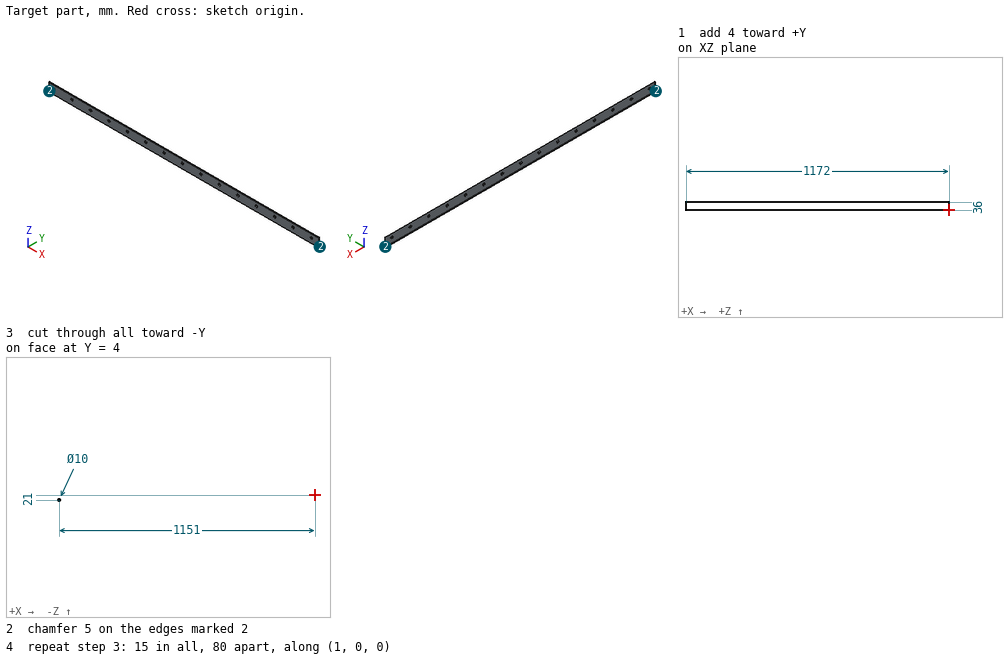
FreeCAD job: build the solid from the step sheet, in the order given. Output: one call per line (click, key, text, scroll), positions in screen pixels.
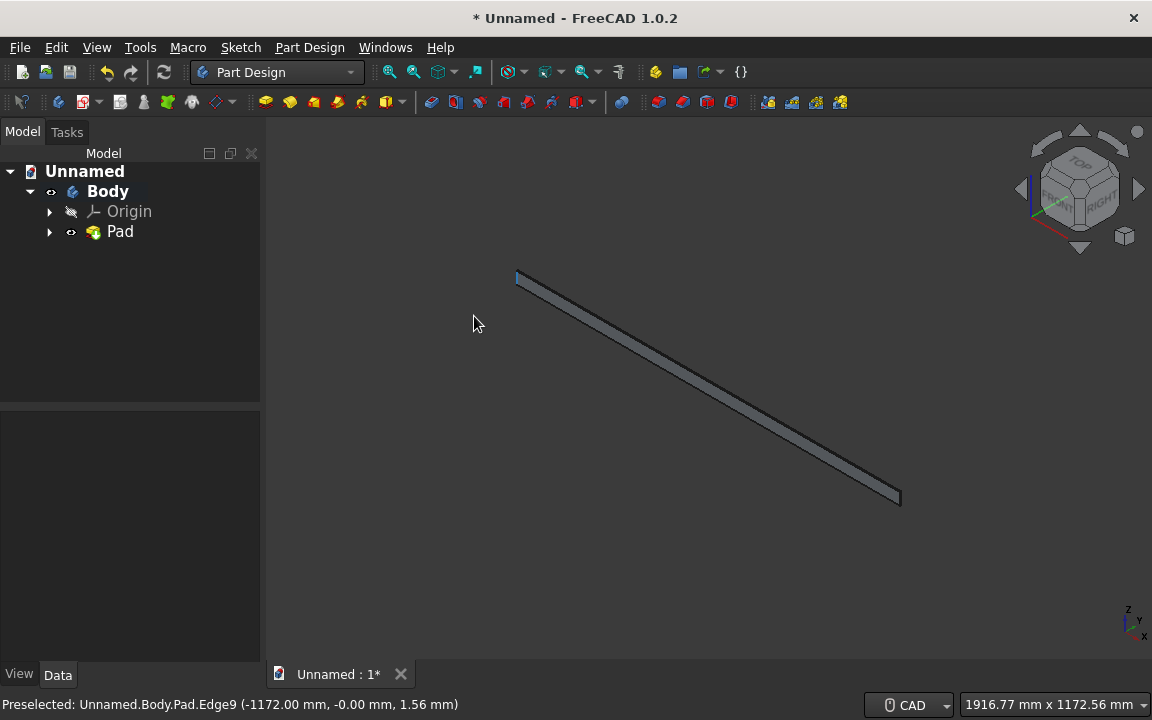
key(v)
key(f)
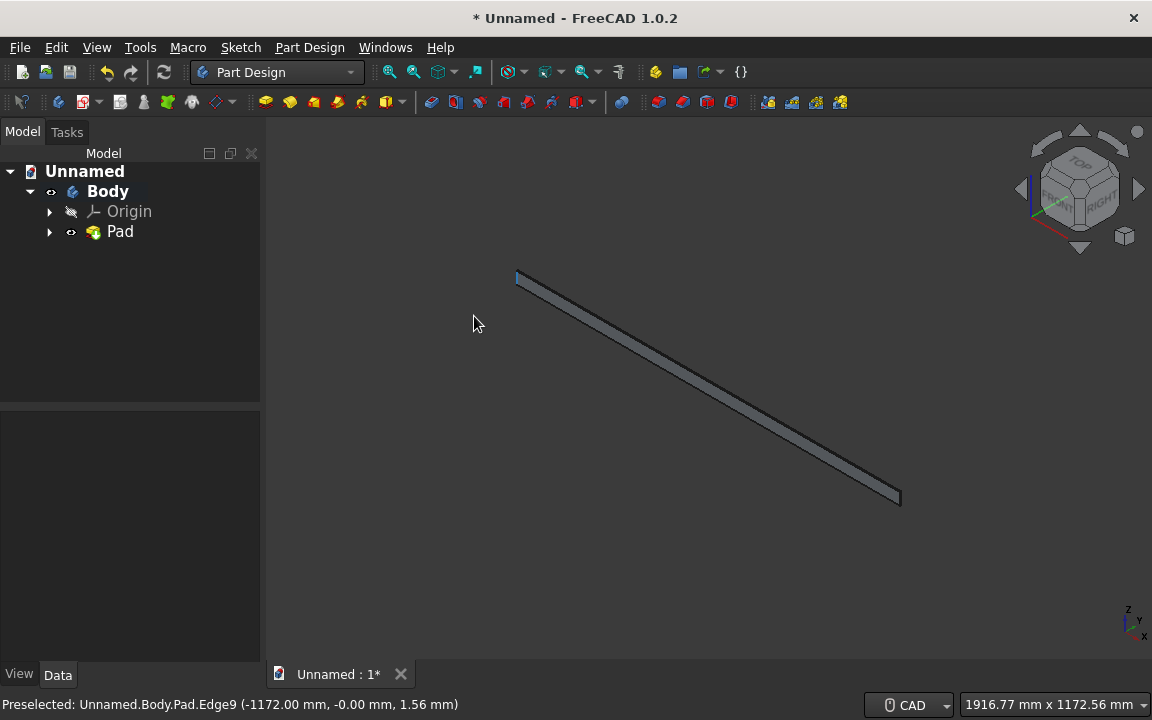
scroll(517, 283, up, 15)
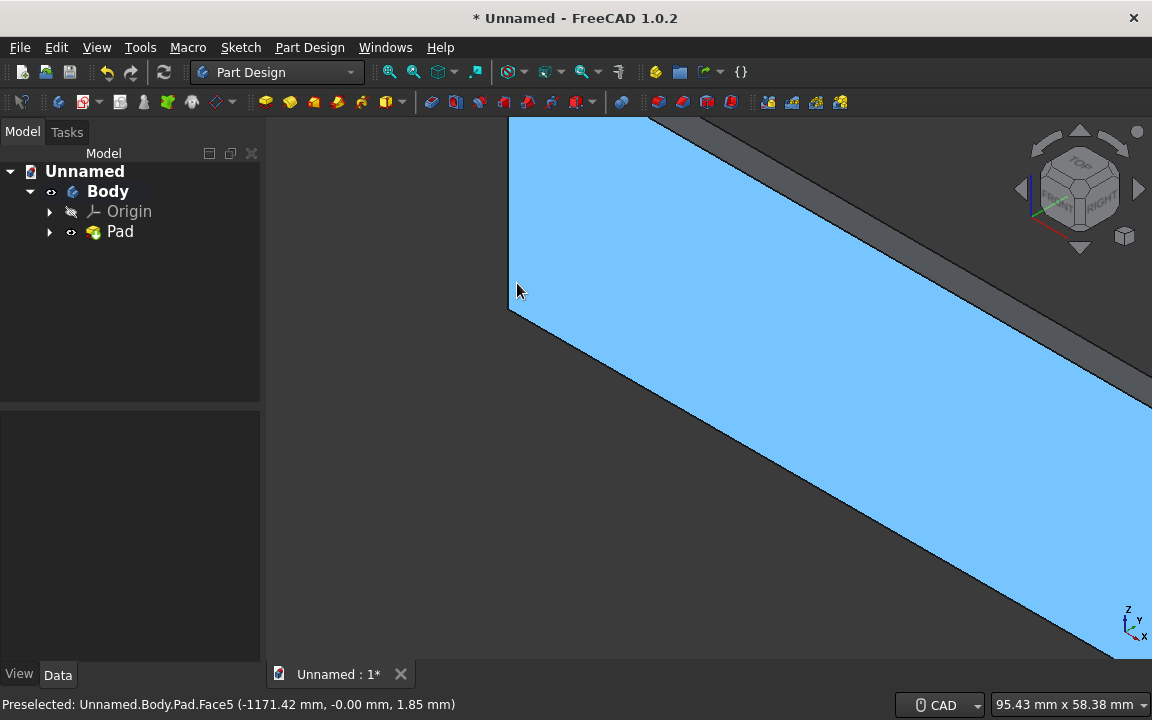
click(390, 72)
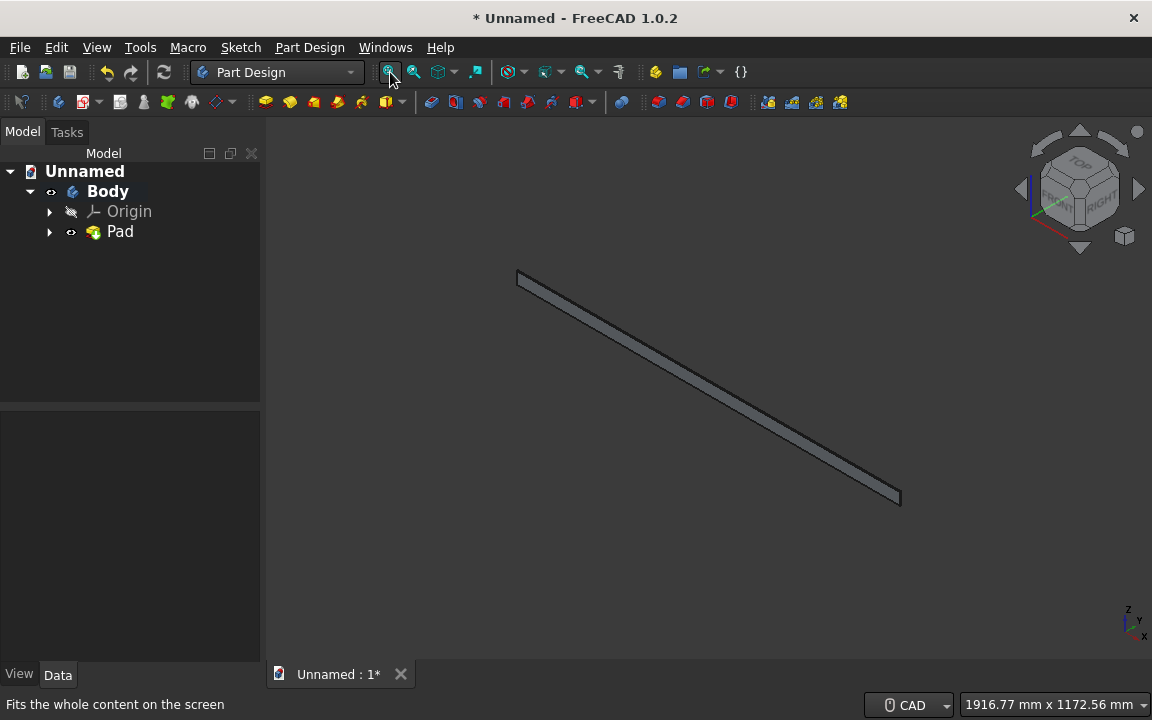
key(2)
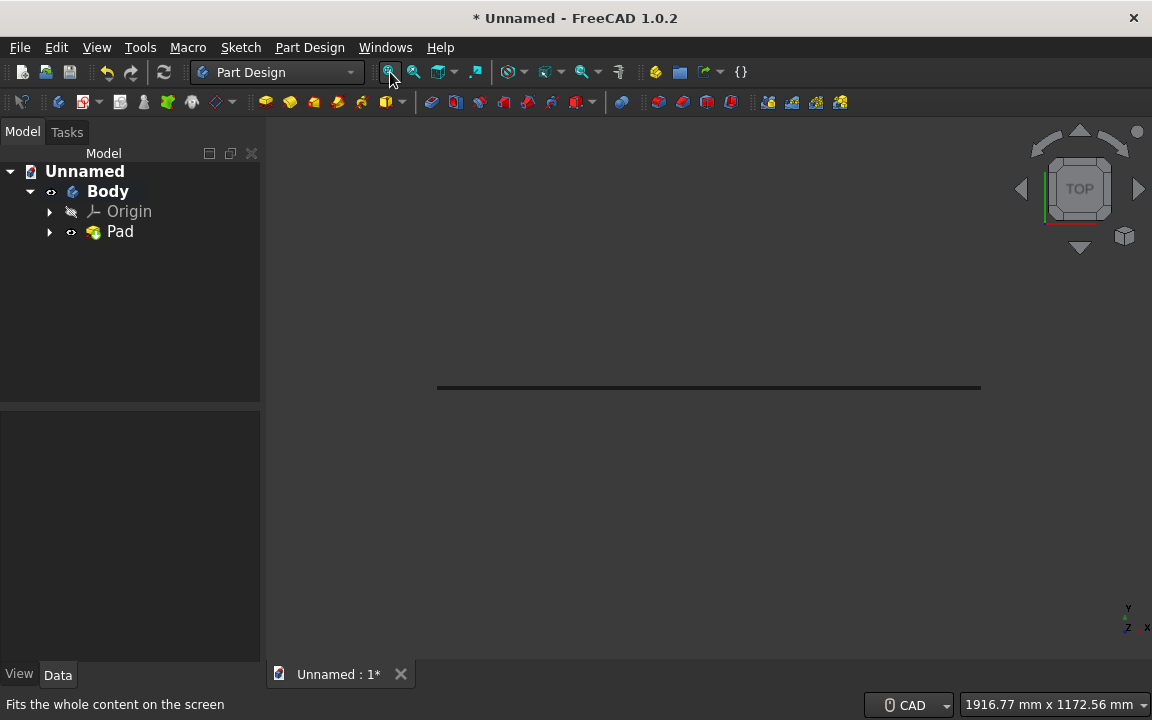
scroll(438, 387, up, 15)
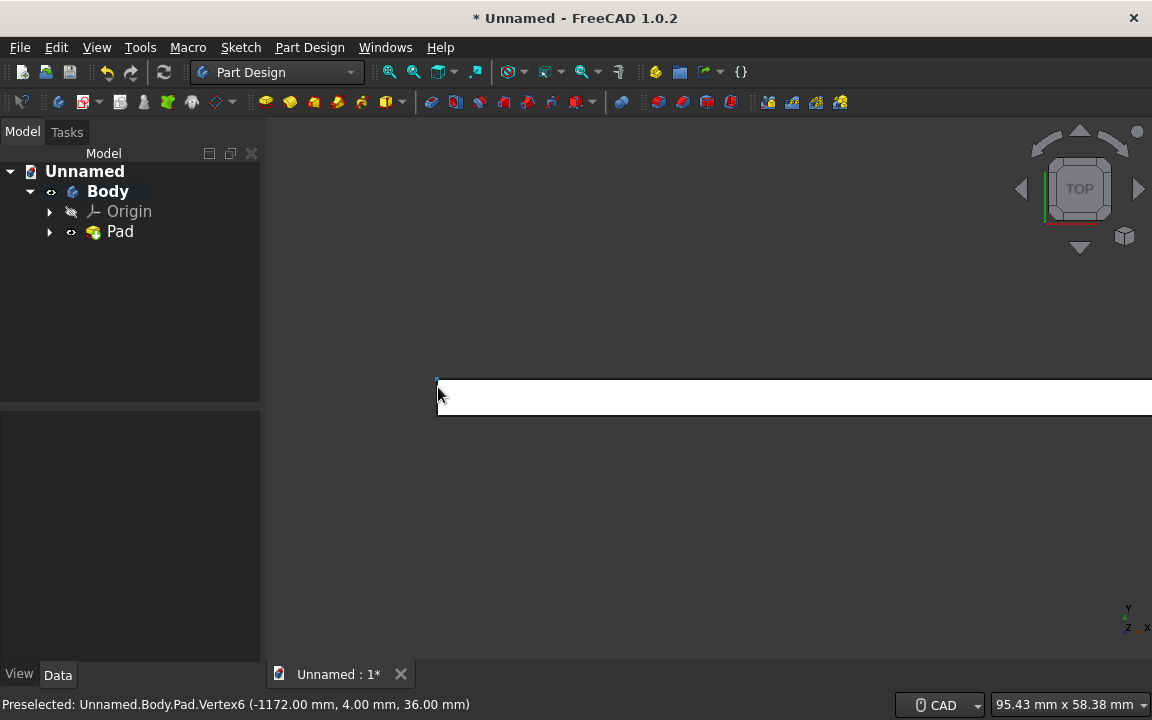
click(390, 72)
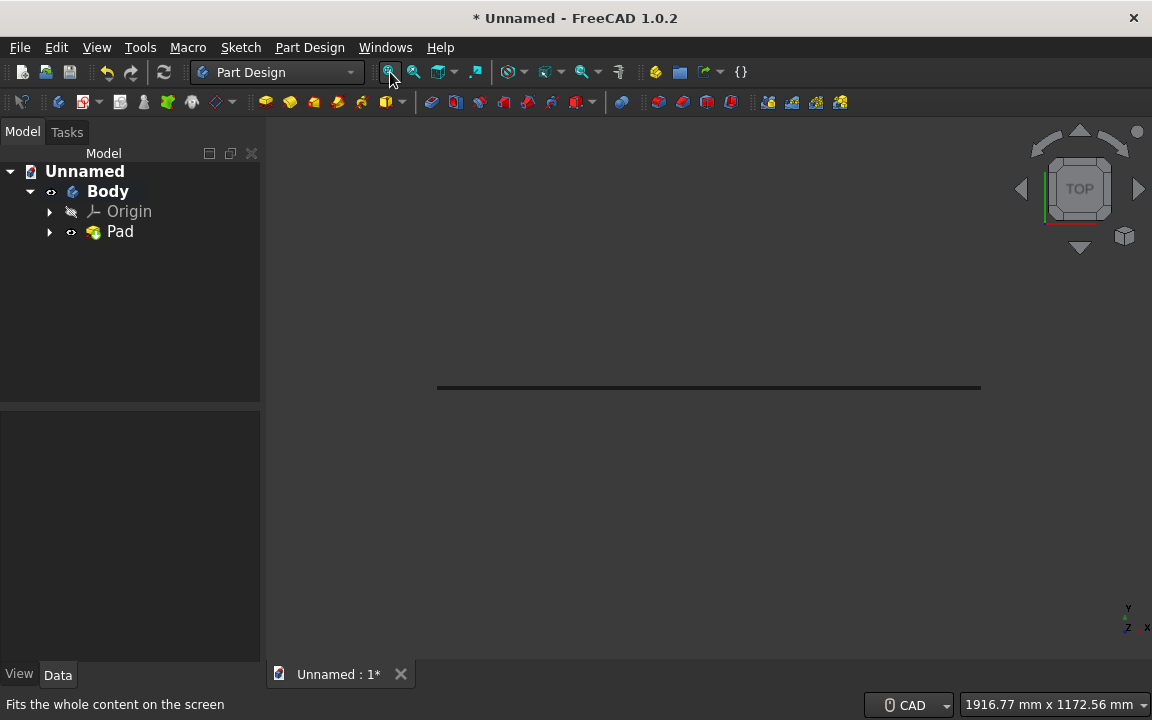
key(1)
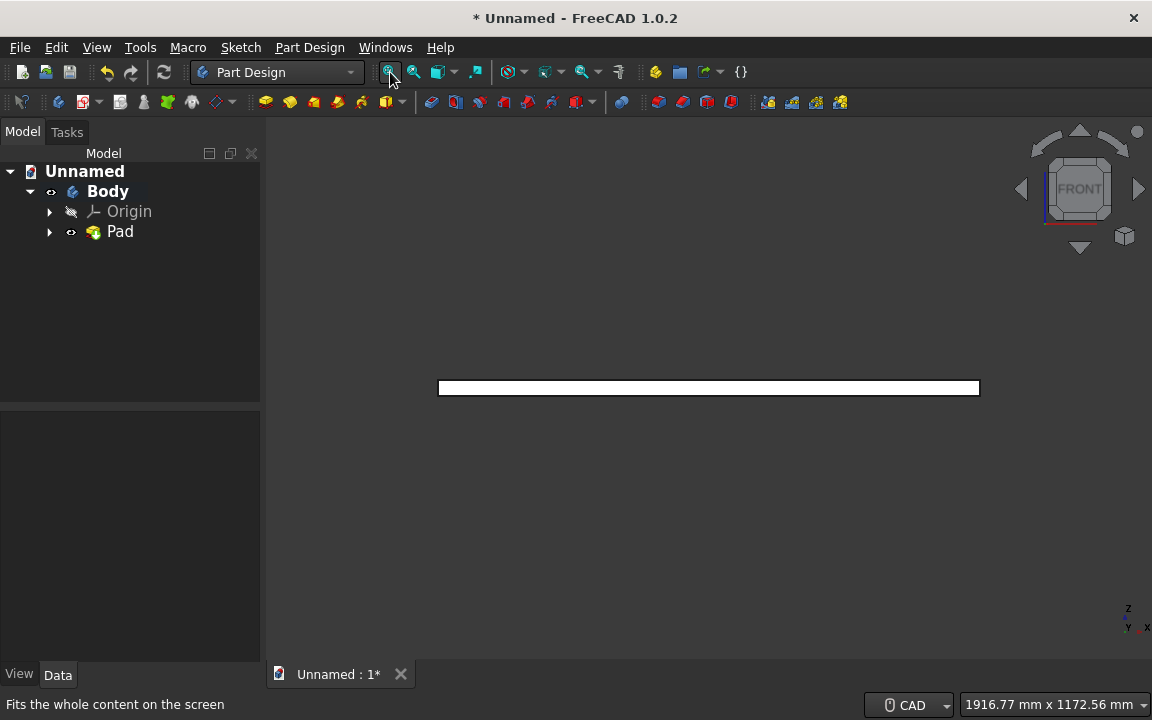
scroll(438, 395, up, 15)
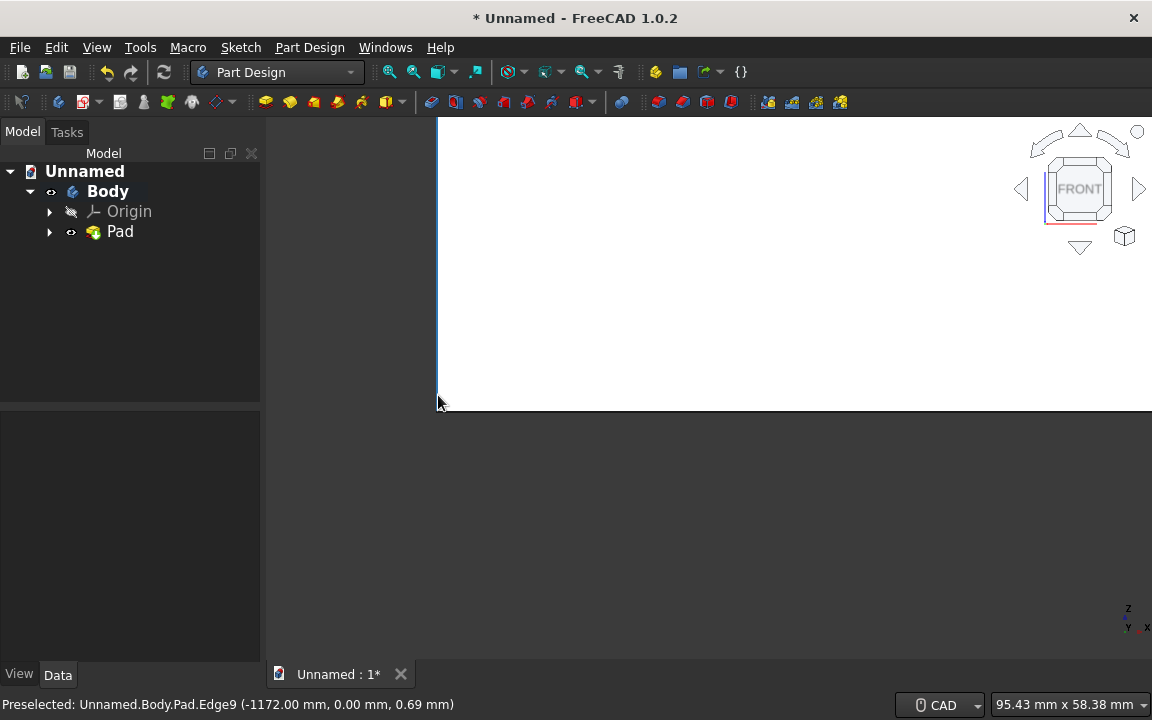
click(390, 72)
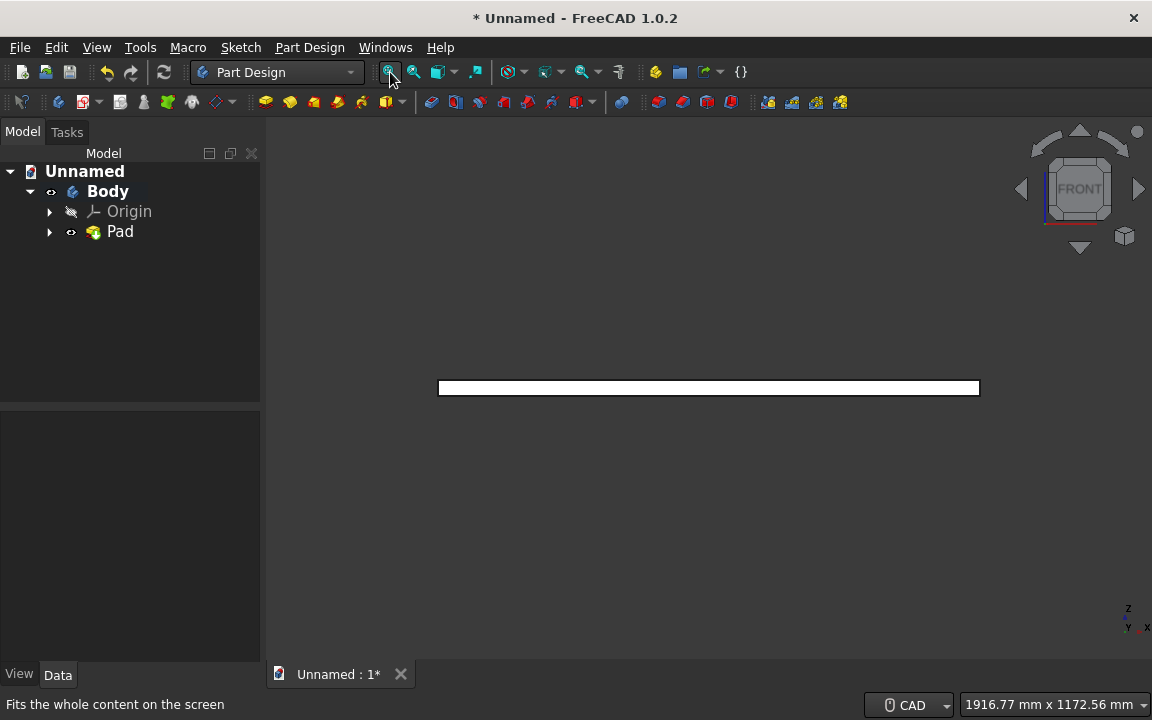
key(3)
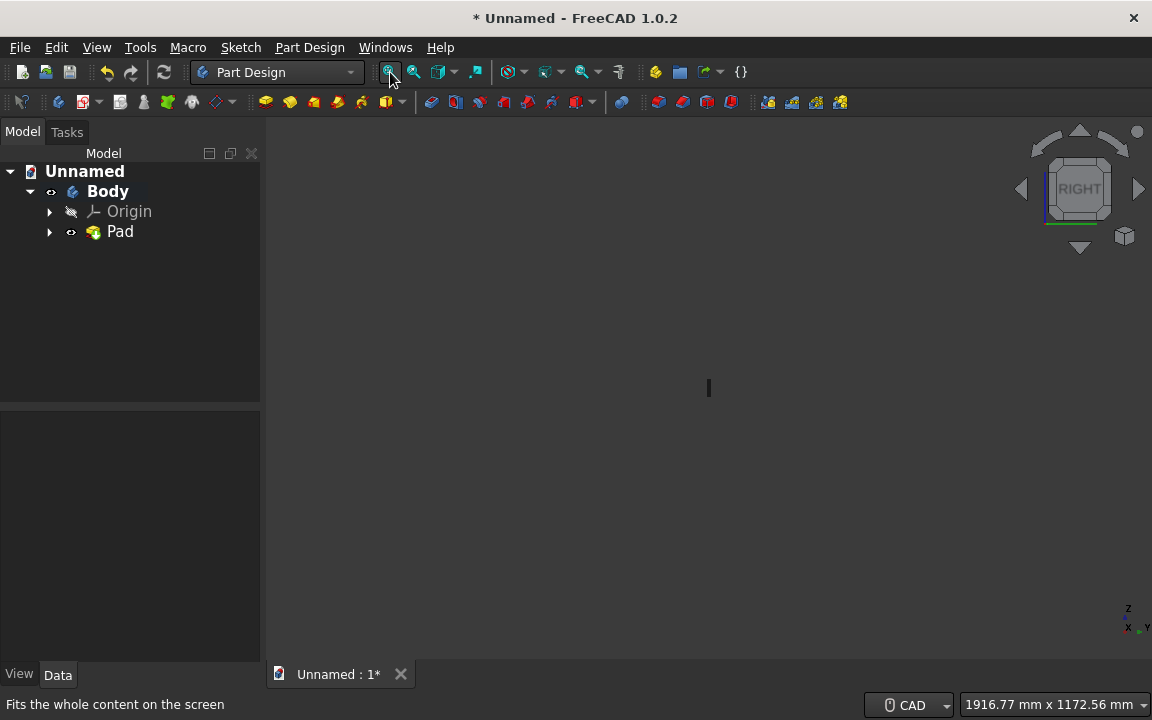
click(390, 72)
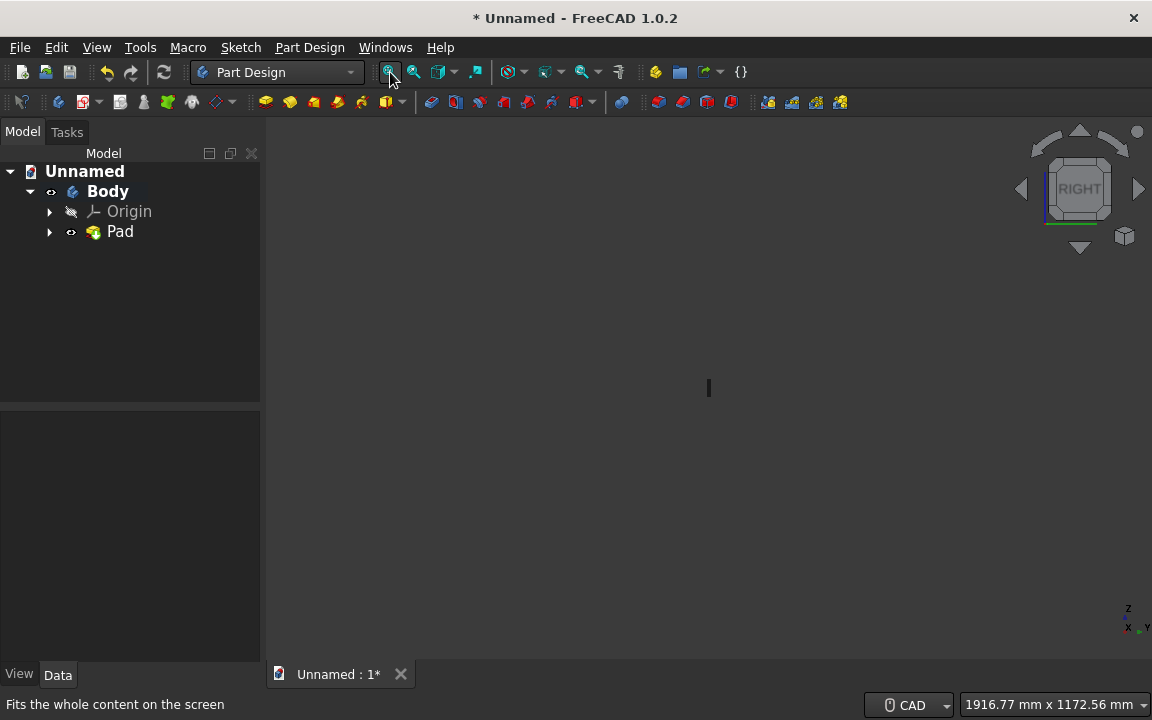
scroll(709, 395, up, 15)